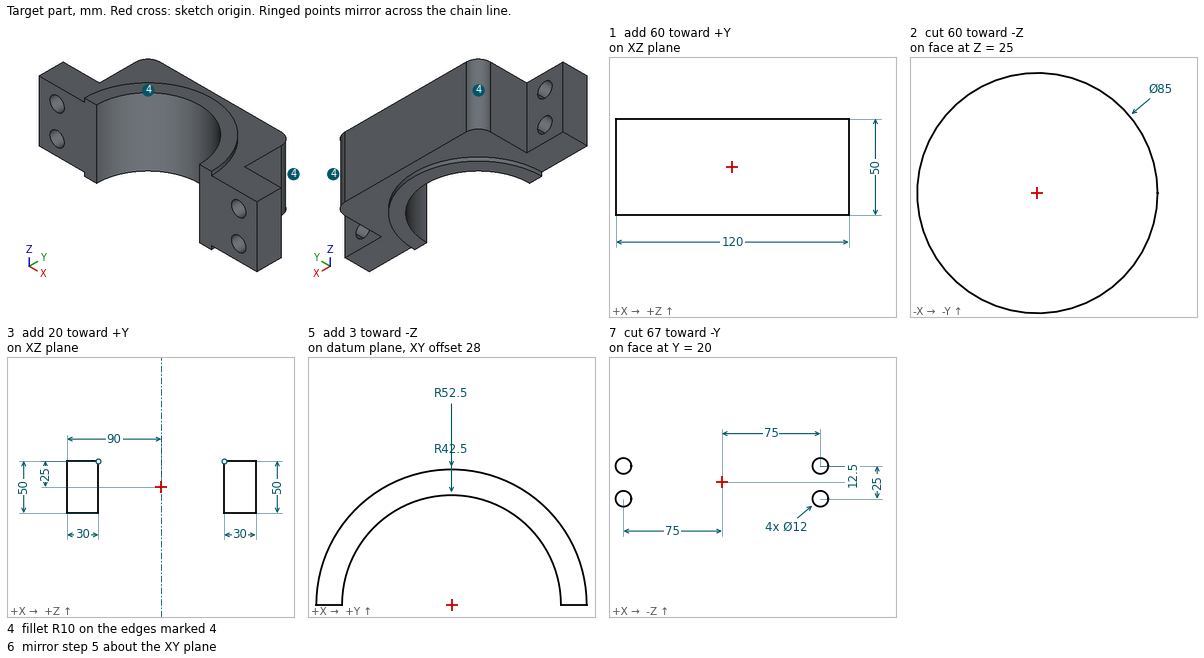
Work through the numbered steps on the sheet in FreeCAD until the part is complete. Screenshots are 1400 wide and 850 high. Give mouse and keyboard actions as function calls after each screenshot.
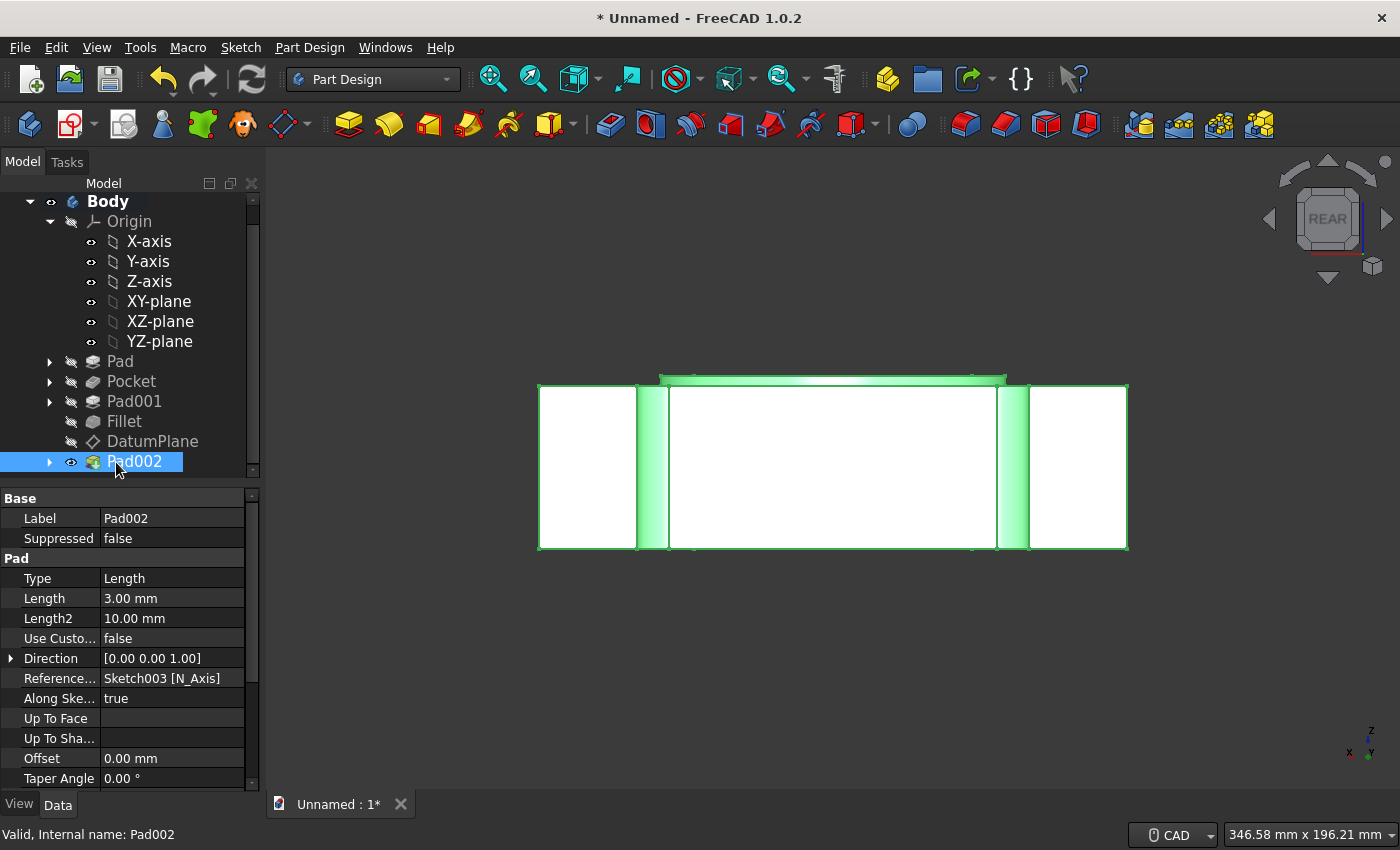
click(1140, 124)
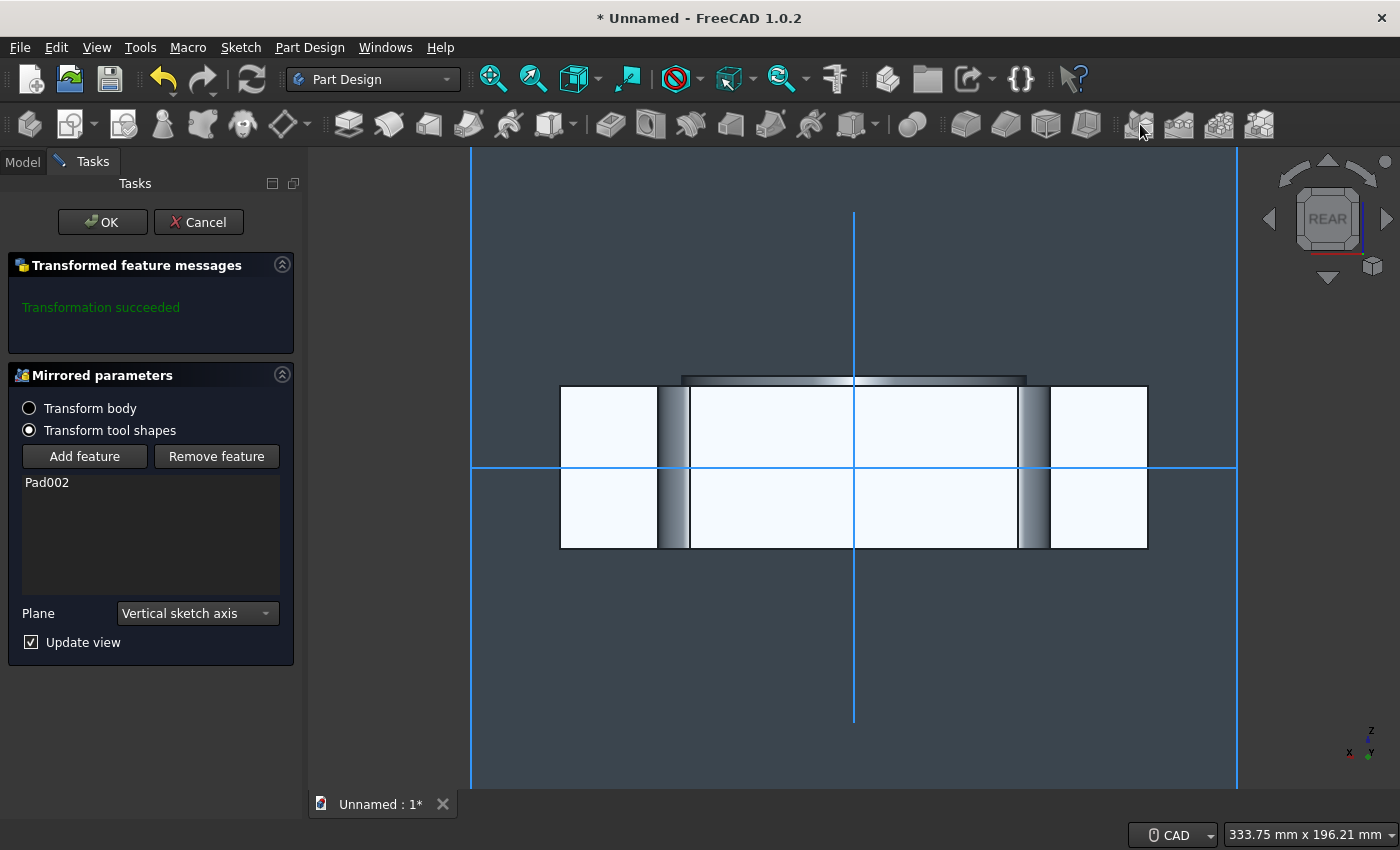
click(198, 614)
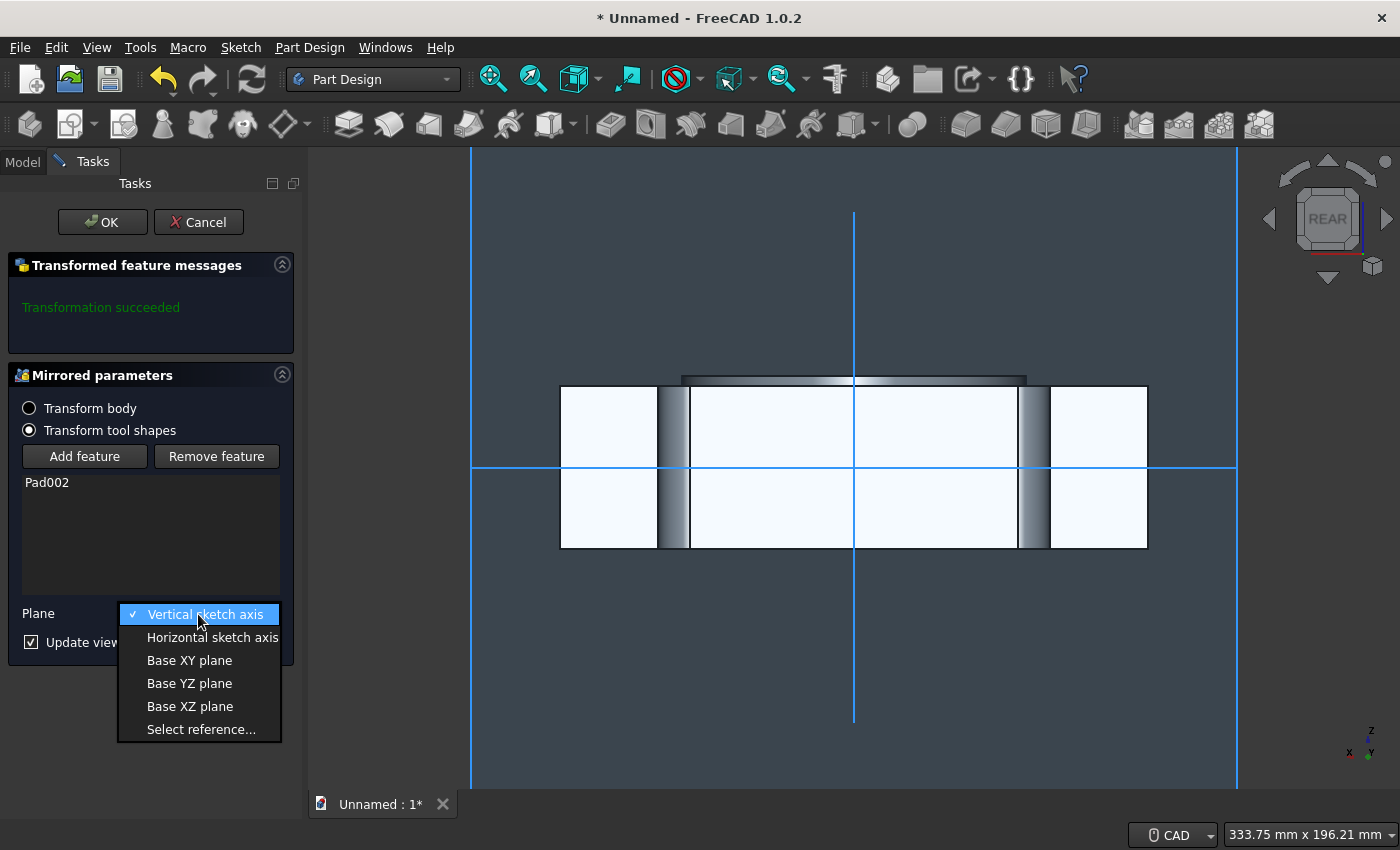
click(198, 660)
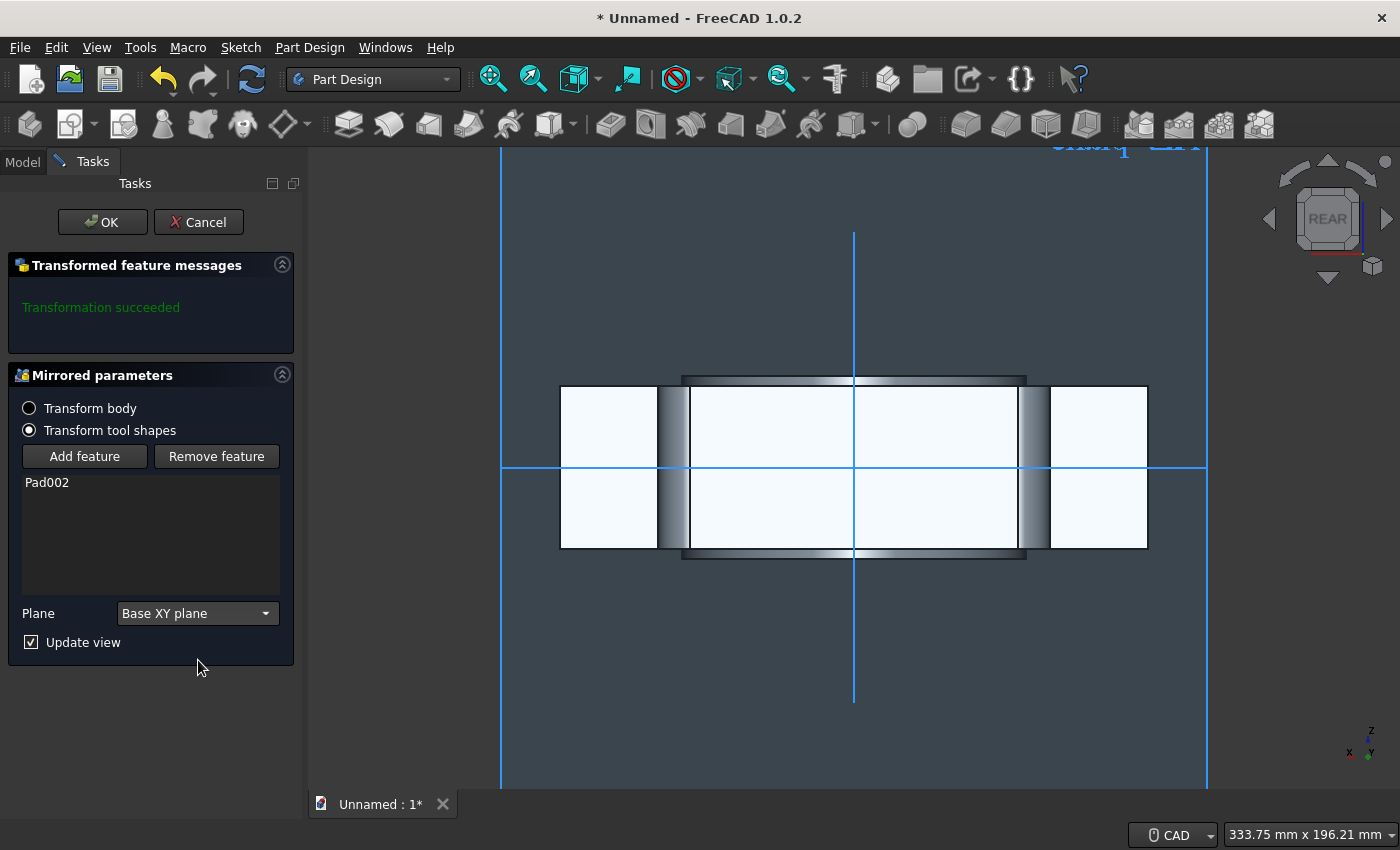
click(103, 222)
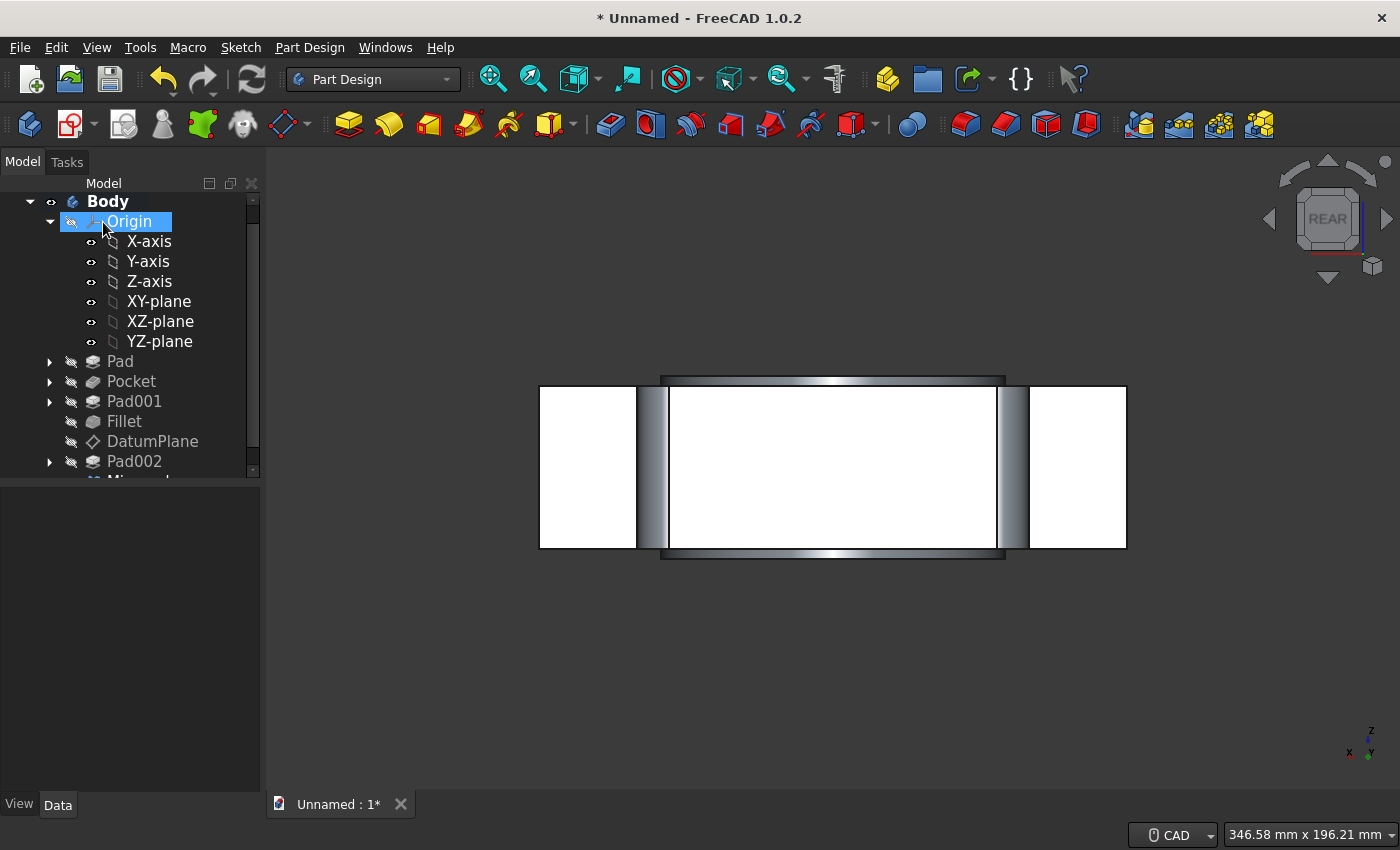
click(1078, 443)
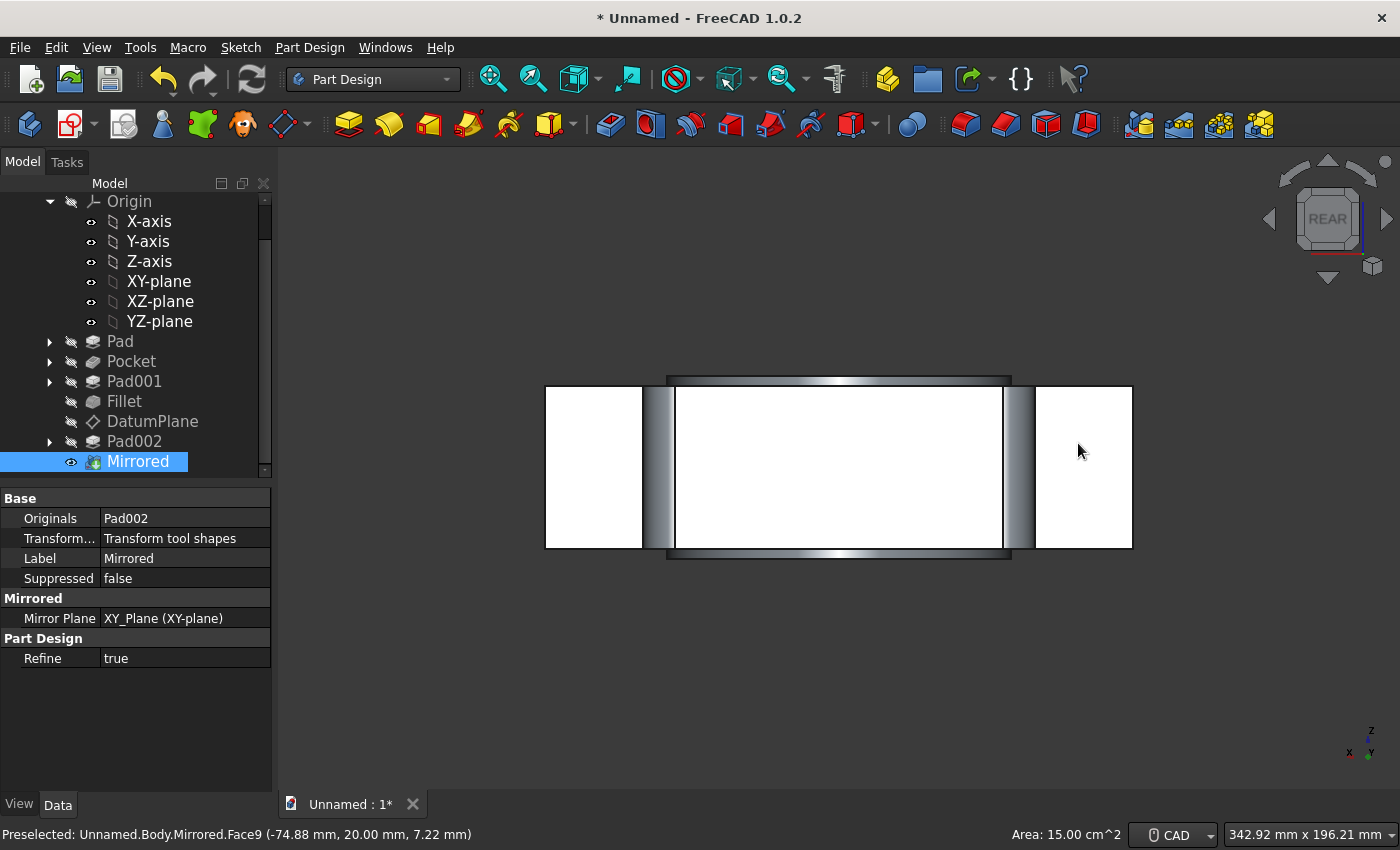
click(70, 124)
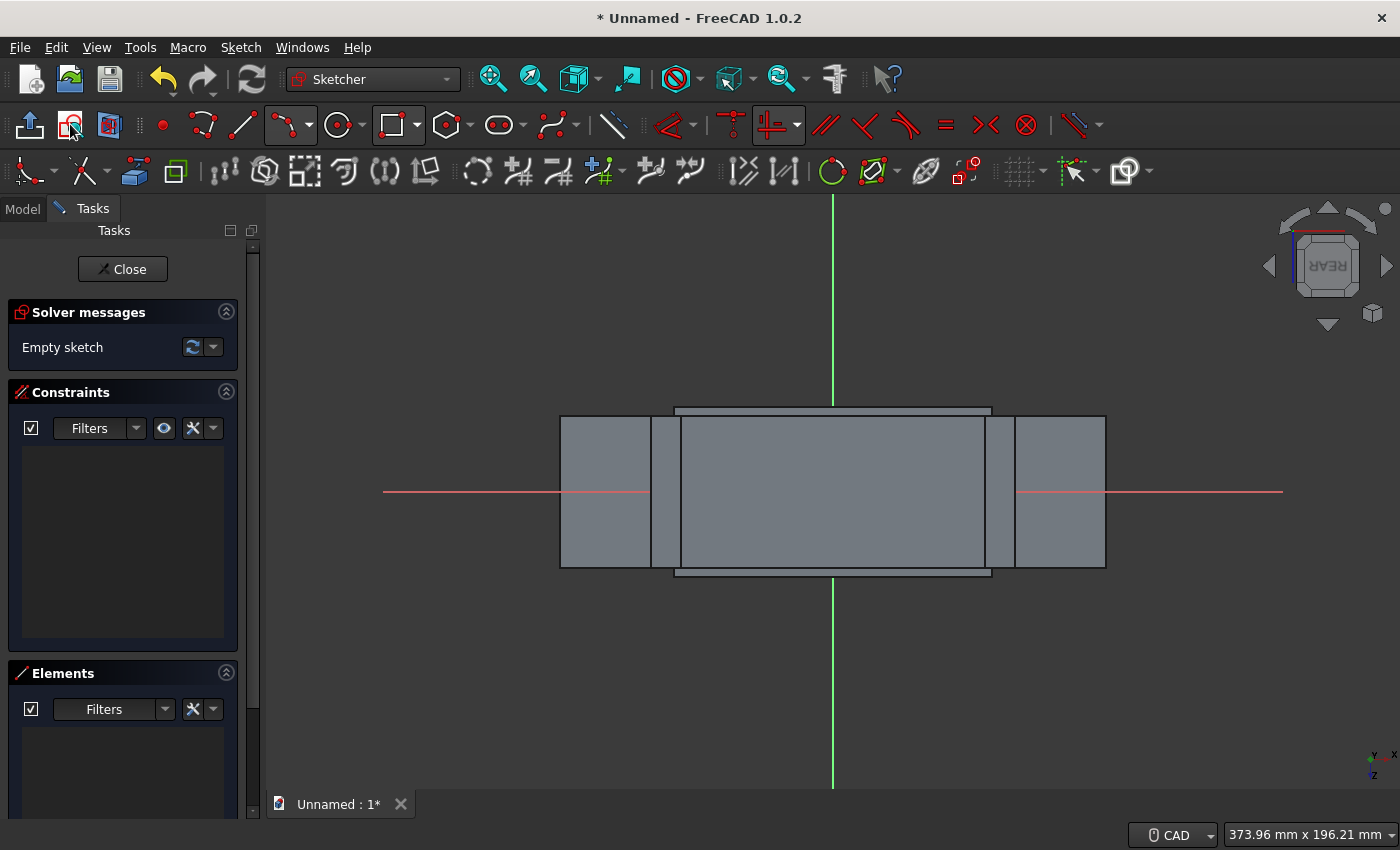
scroll(972, 493, up, 2)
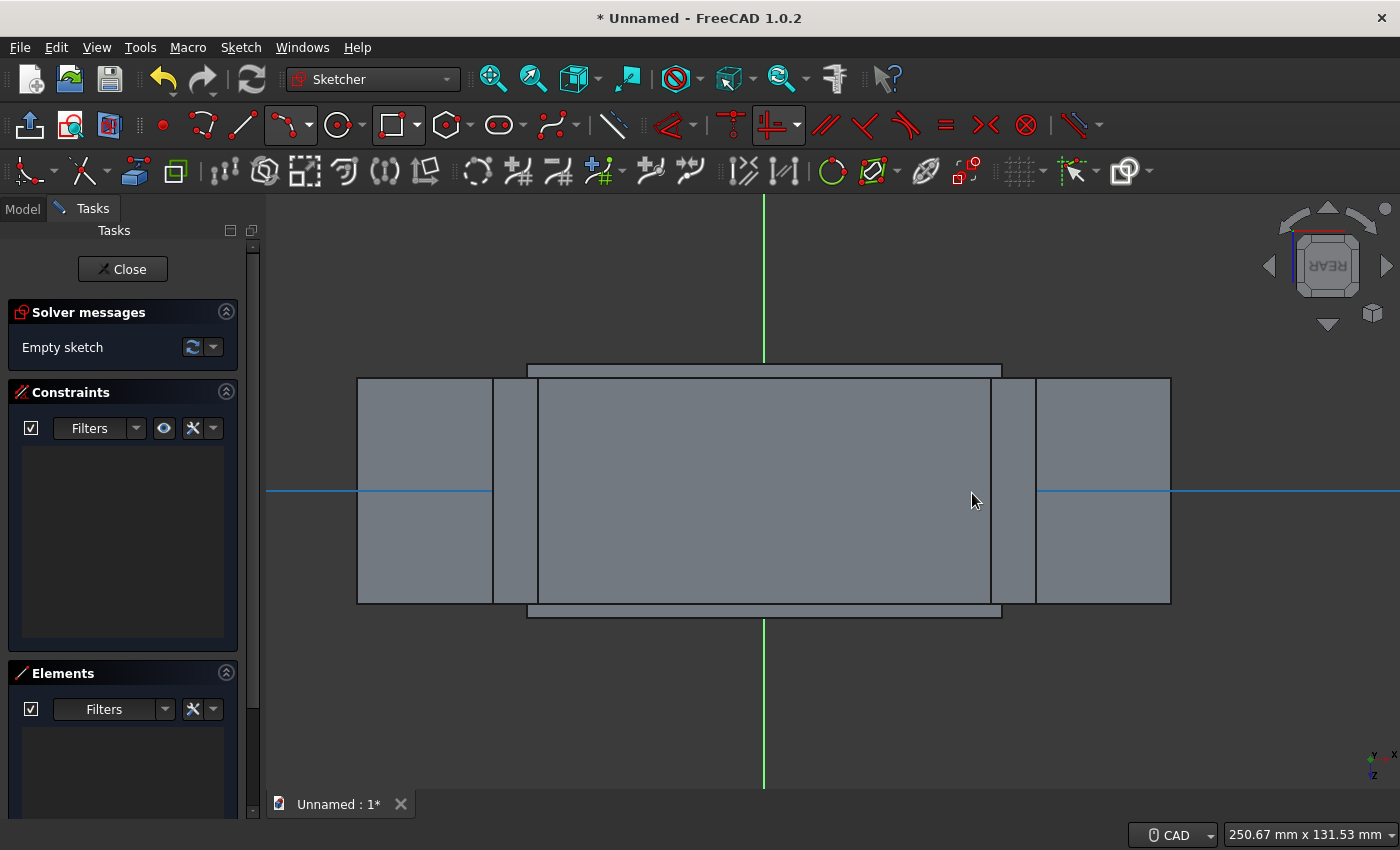
click(338, 126)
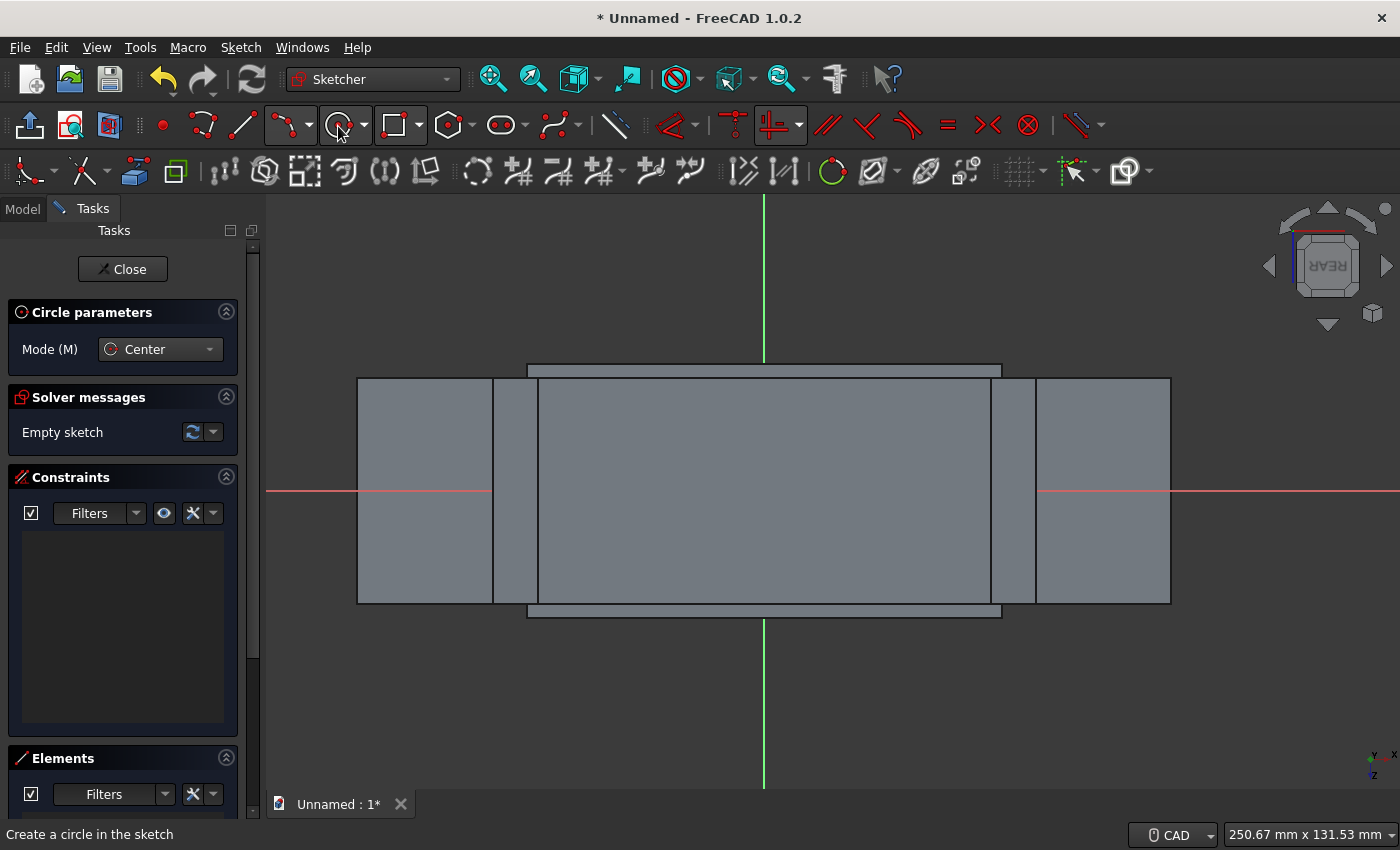
click(1104, 434)
move(1123, 415)